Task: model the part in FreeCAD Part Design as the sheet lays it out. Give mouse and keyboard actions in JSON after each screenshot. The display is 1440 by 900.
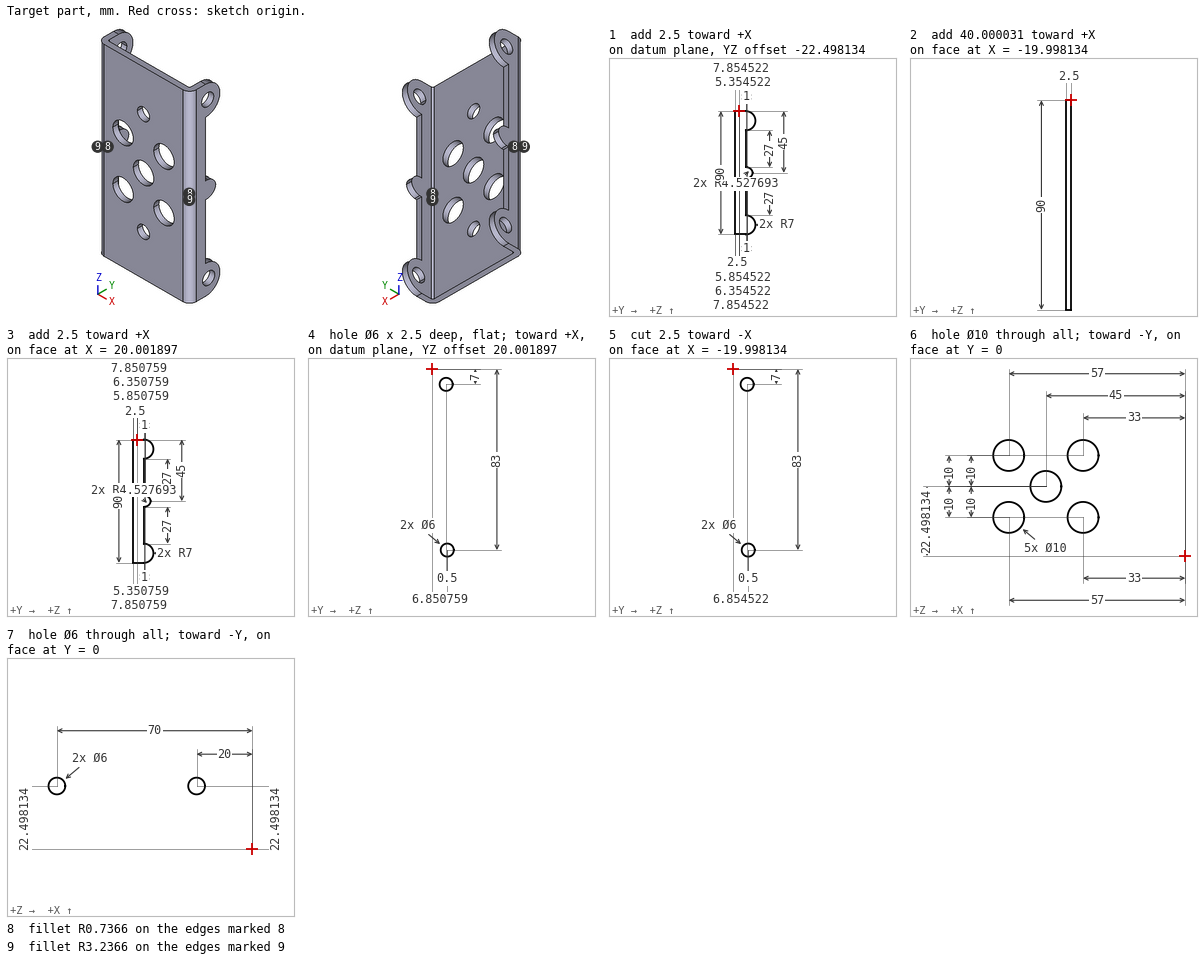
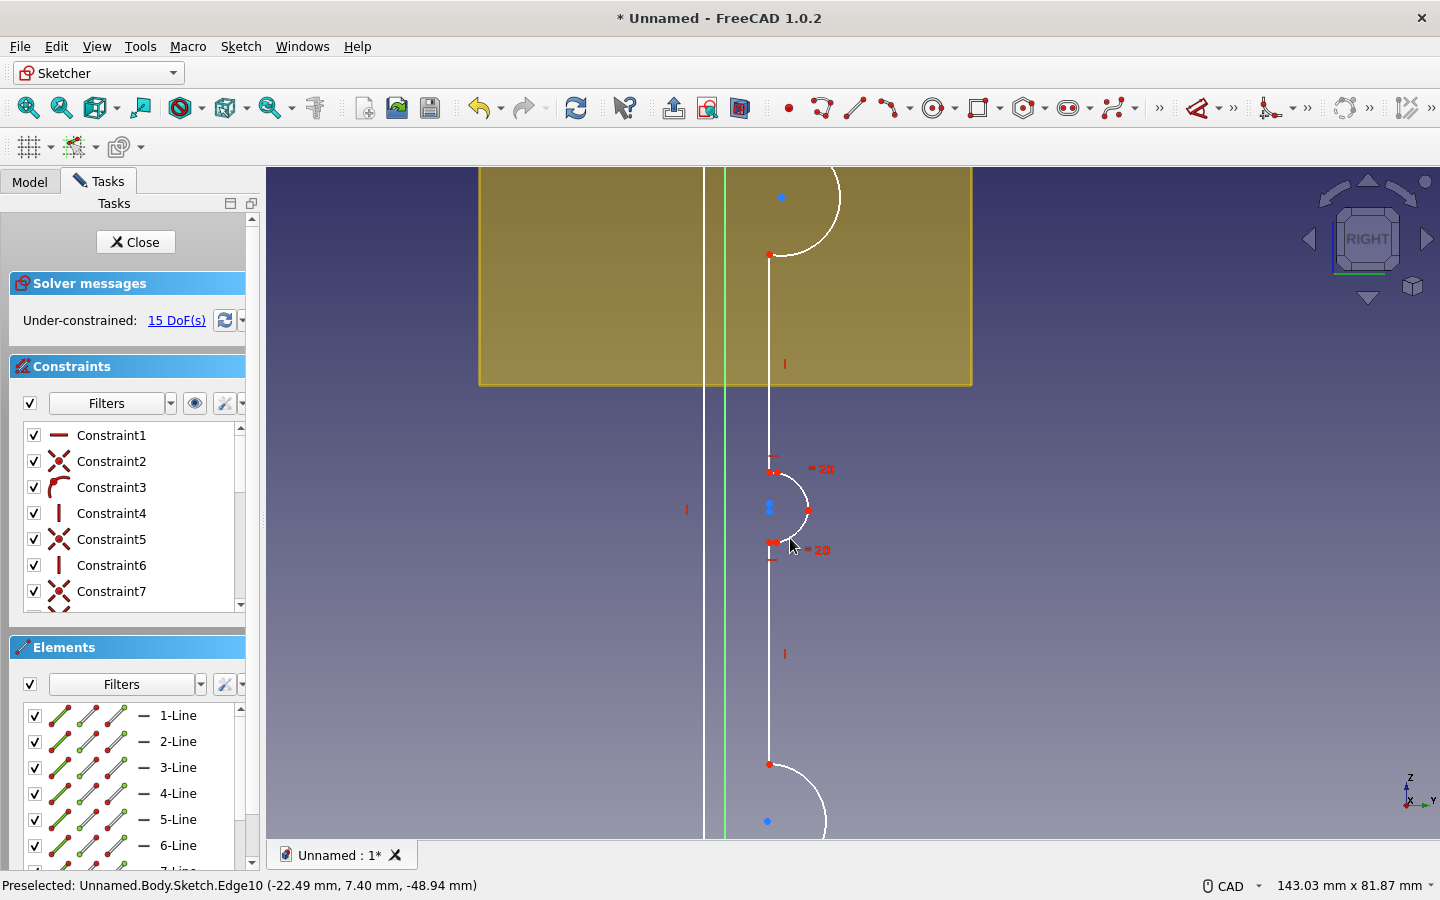
{"action": "left_click", "coordinate": [823, 238]}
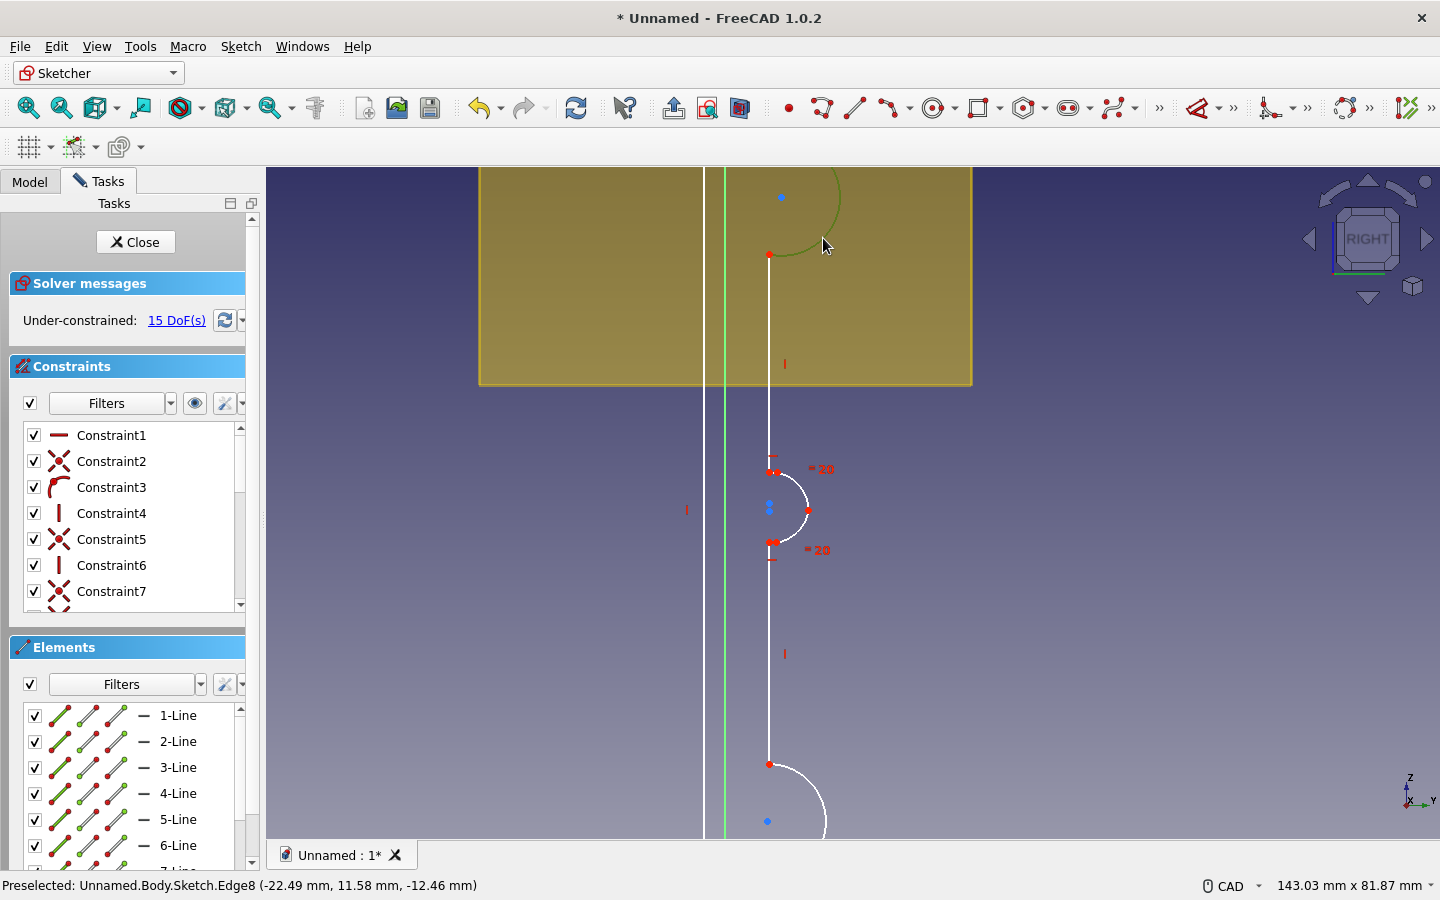
{"action": "left_click", "coordinate": [815, 789]}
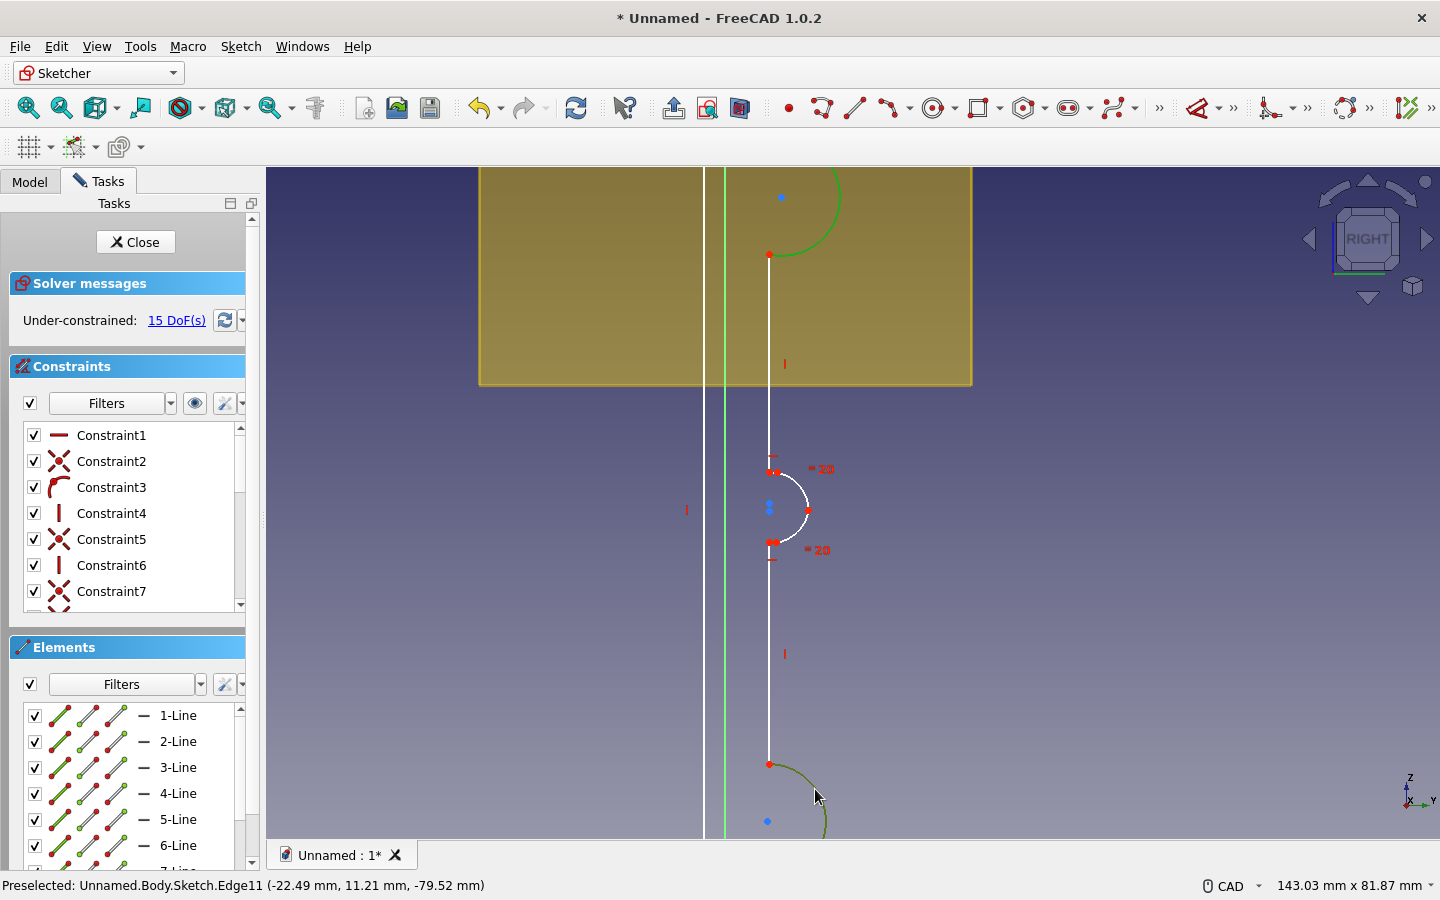
{"action": "key", "text": "e"}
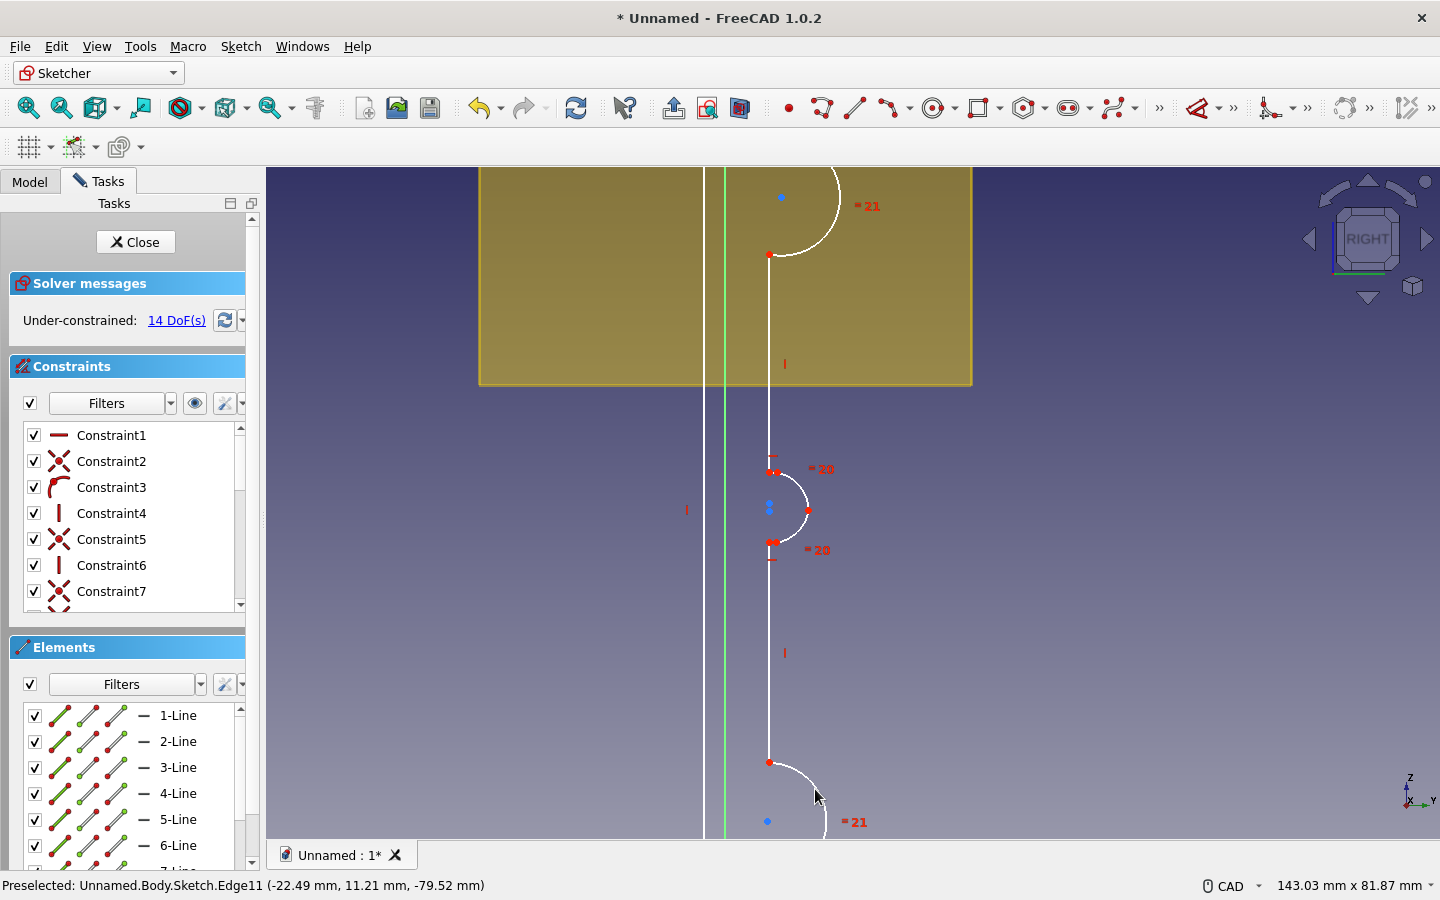
{"action": "left_click", "coordinate": [823, 238]}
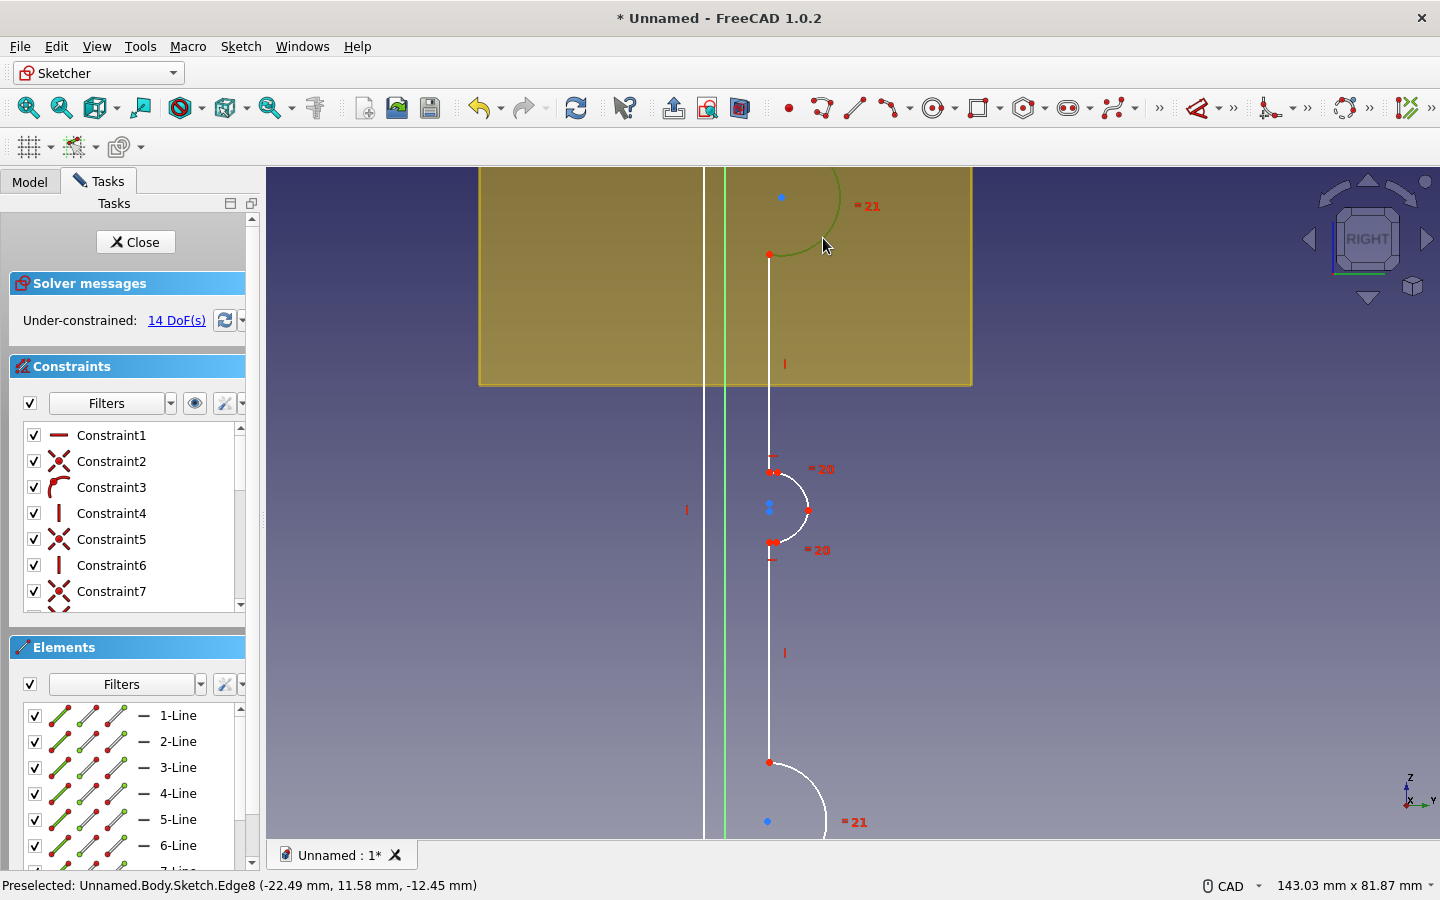
{"action": "key", "text": "k r"}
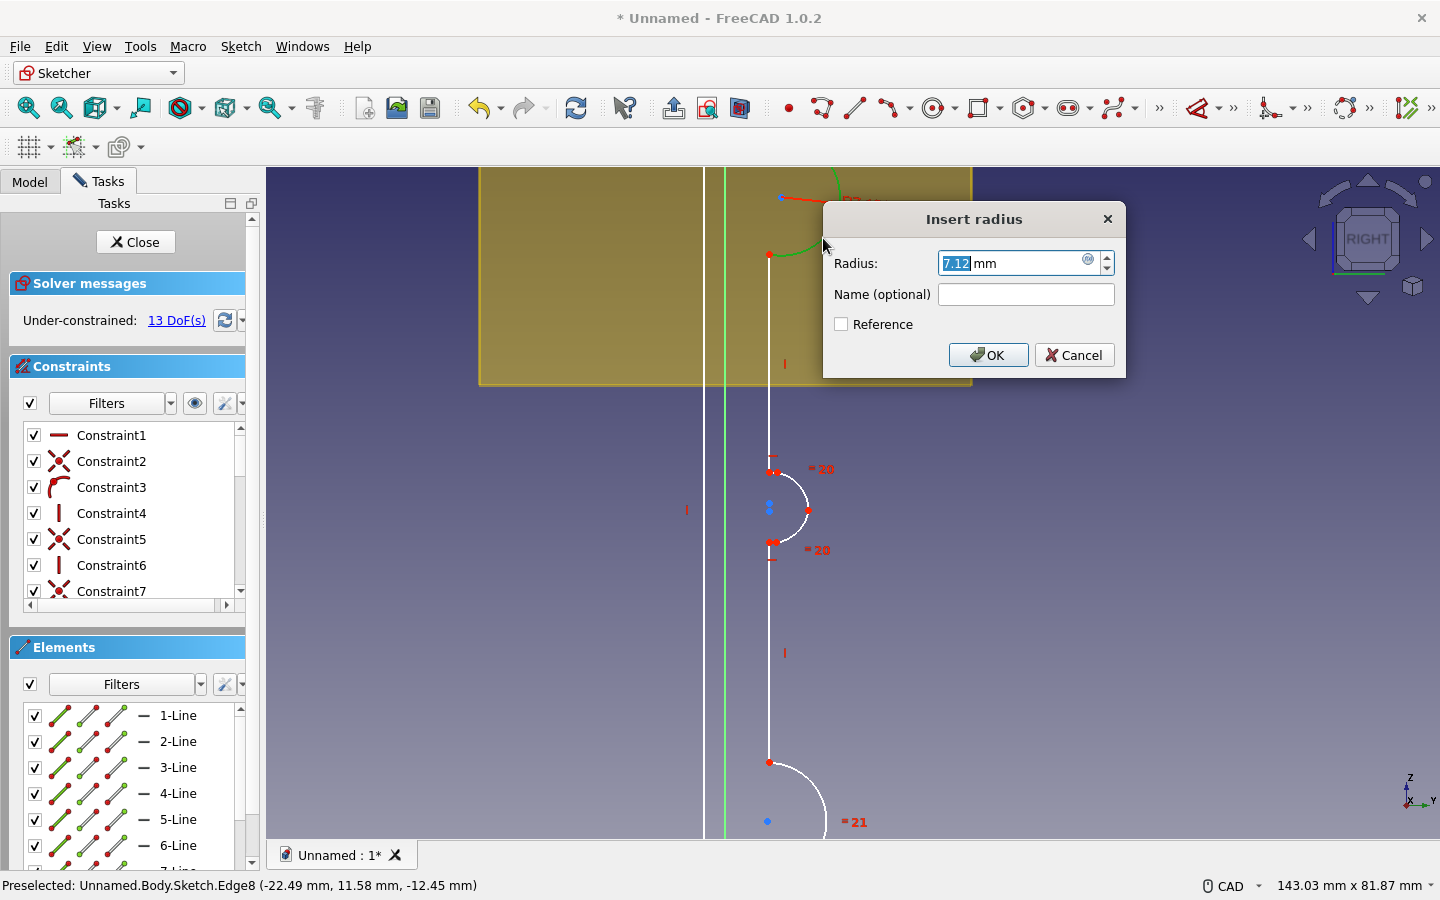
{"action": "type", "text": "7"}
{"action": "key", "text": "Return"}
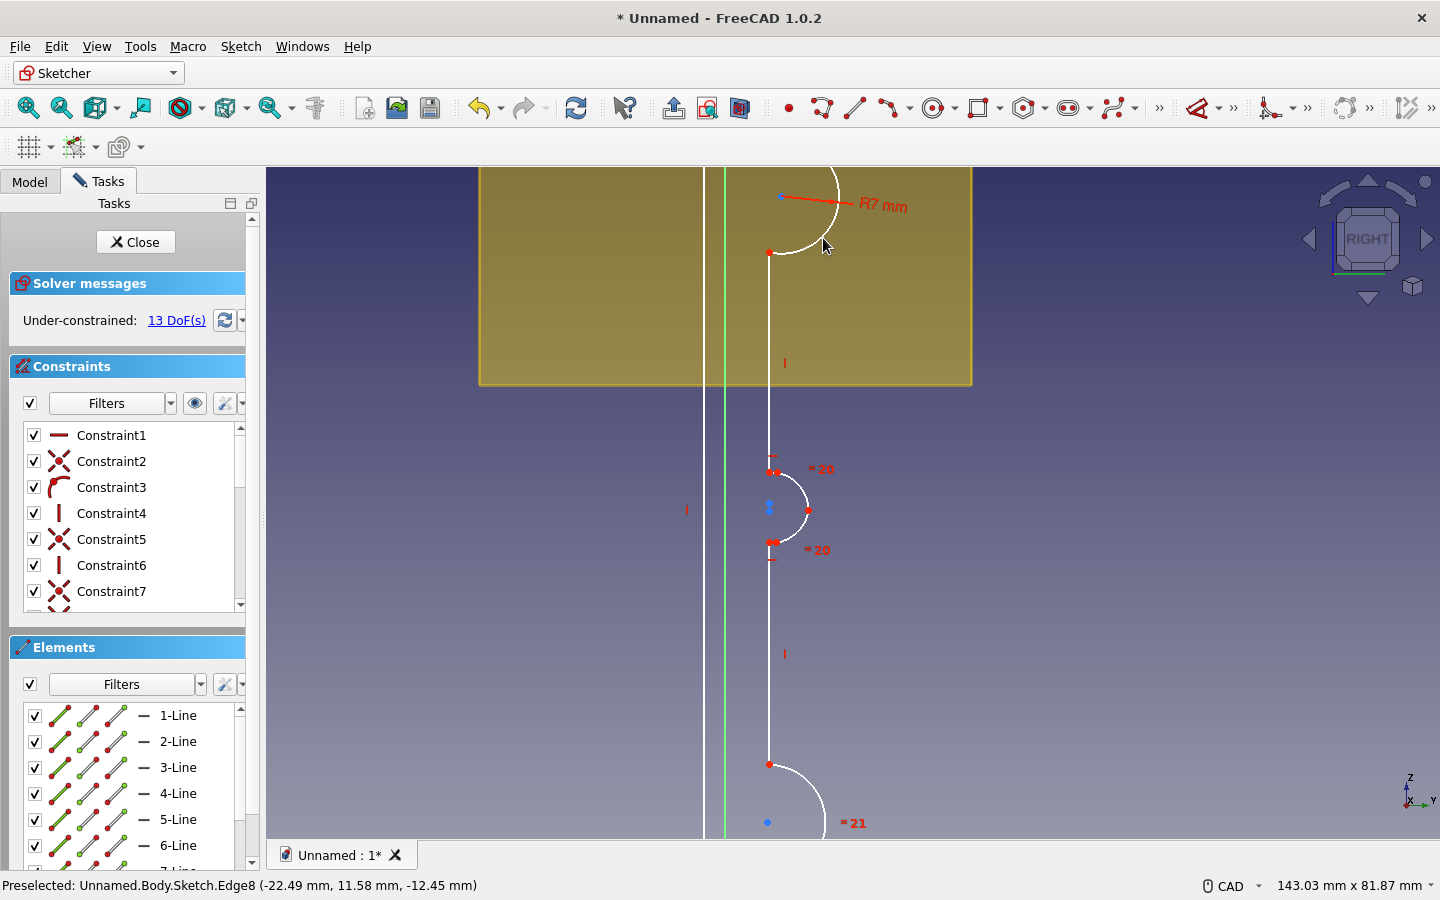
{"action": "left_click", "coordinate": [805, 495]}